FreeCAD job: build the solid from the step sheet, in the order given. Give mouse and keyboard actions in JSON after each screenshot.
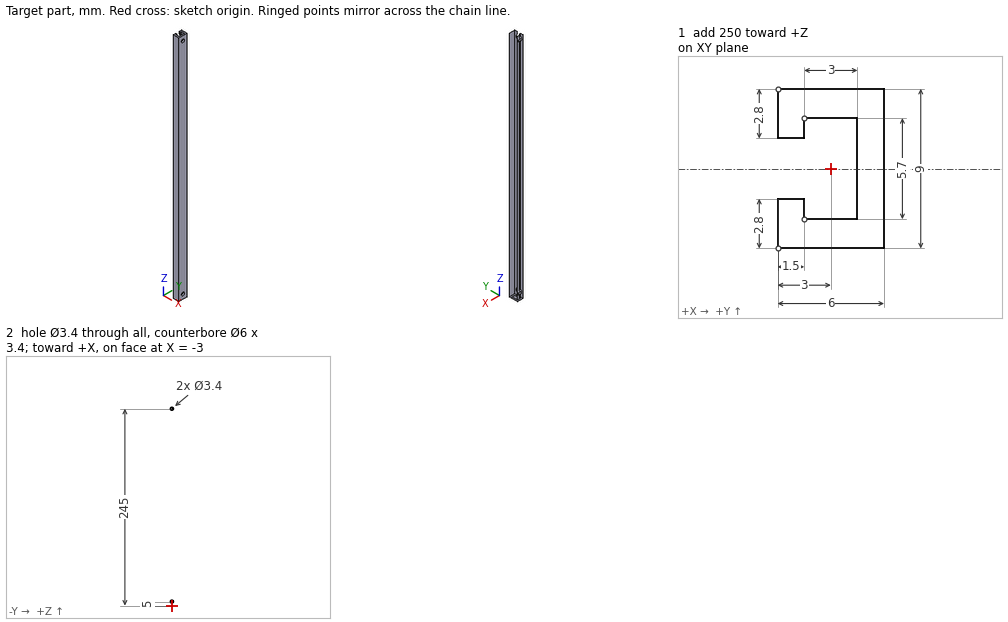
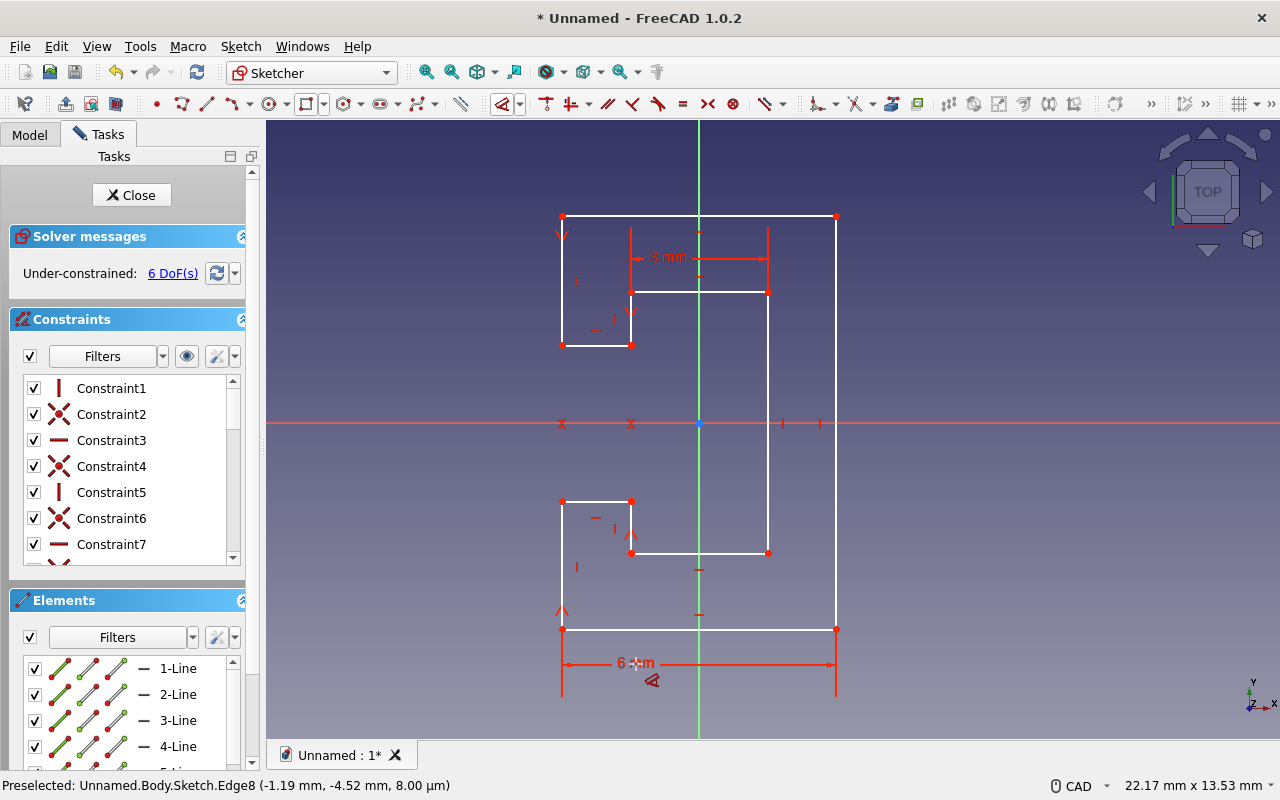
{"action": "left_click", "coordinate": [836, 506]}
{"action": "left_click", "coordinate": [870, 328]}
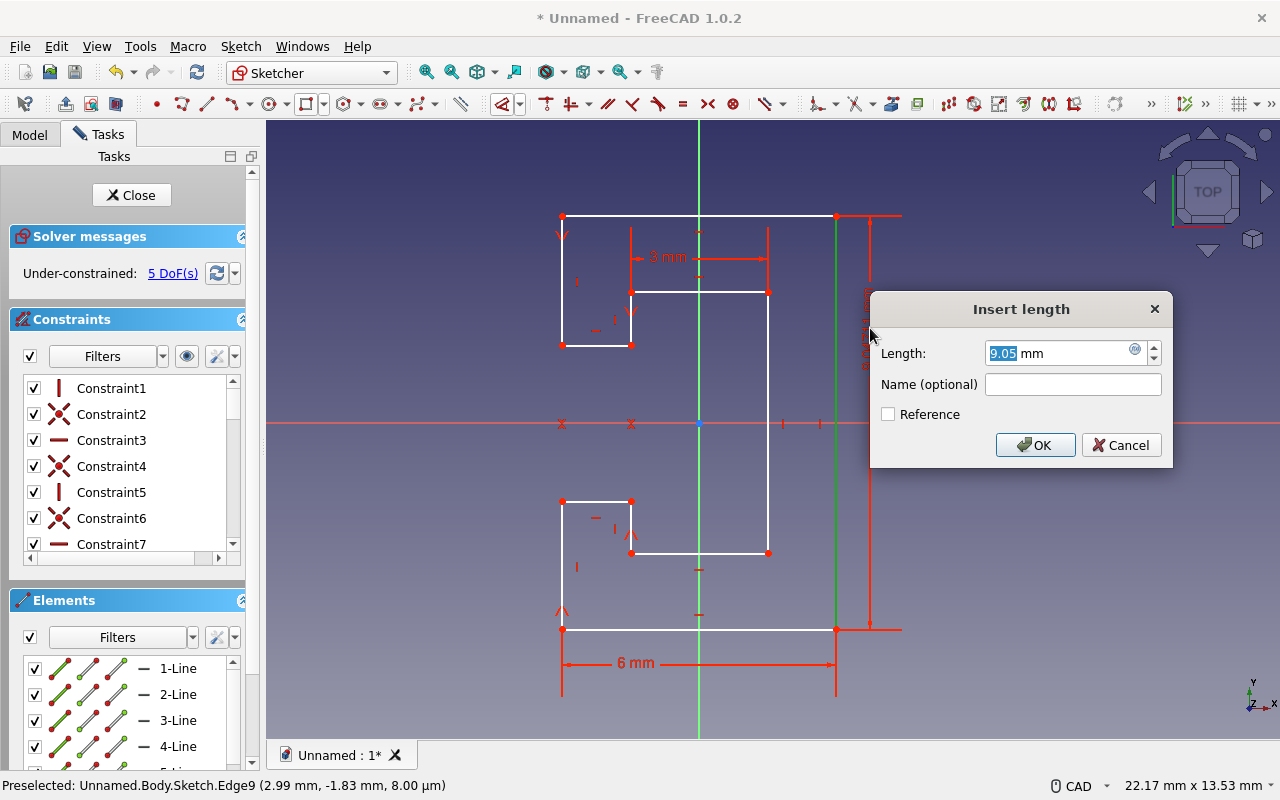
{"action": "type", "text": "9"}
{"action": "key", "text": "Return"}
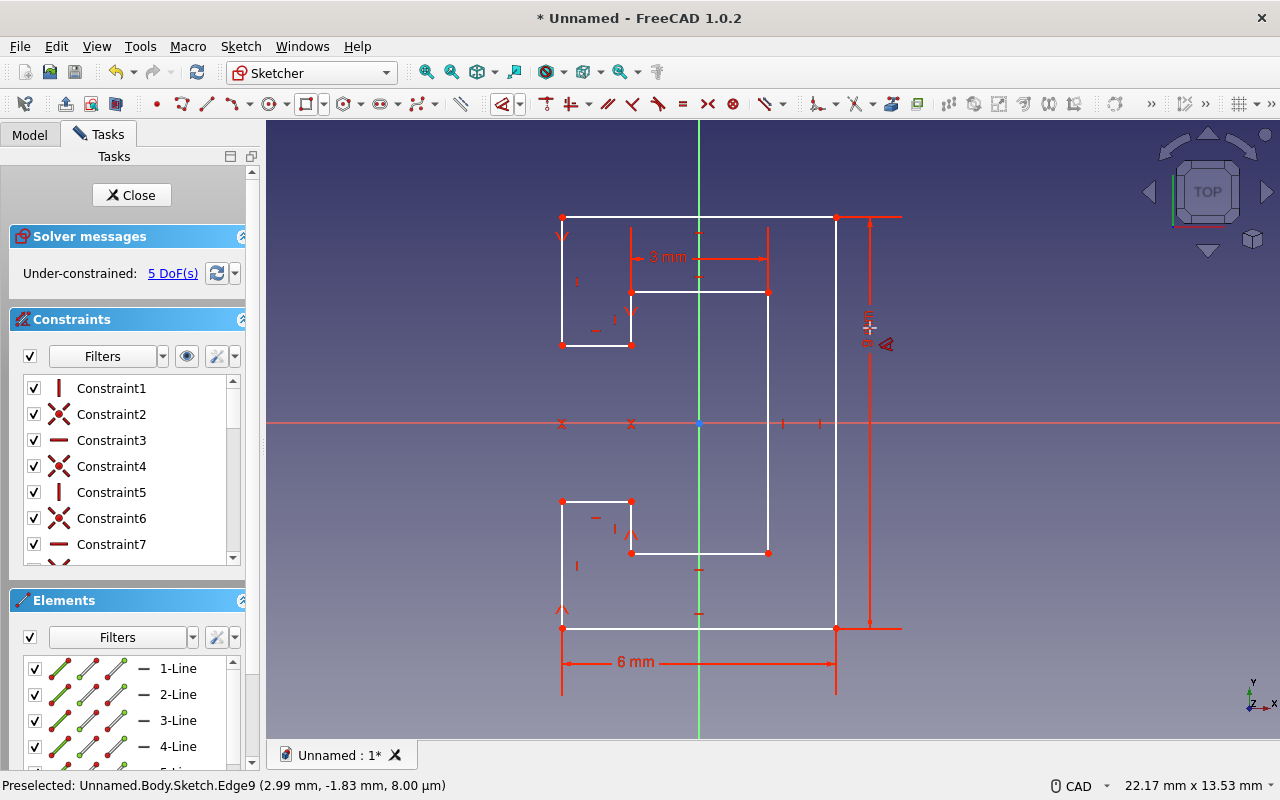
{"action": "left_click", "coordinate": [562, 502]}
{"action": "left_click", "coordinate": [599, 536]}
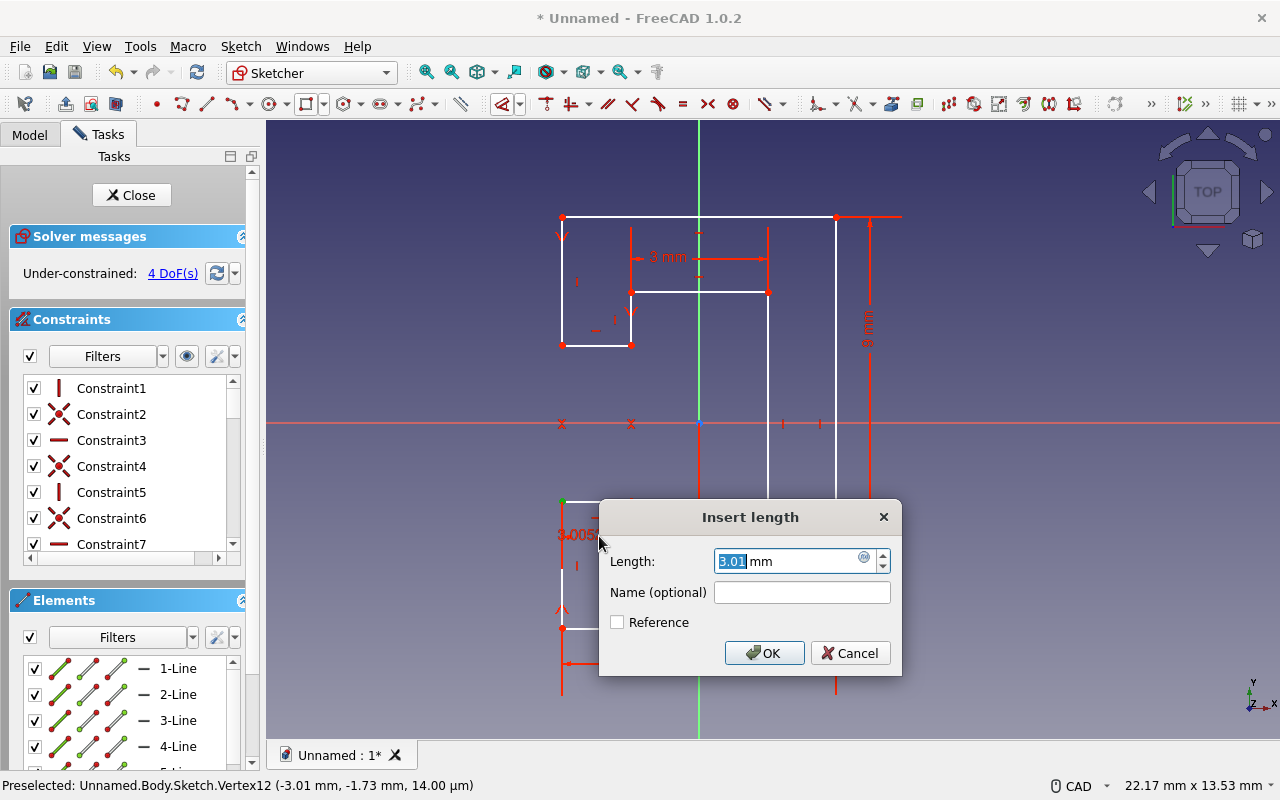
{"action": "type", "text": "3"}
{"action": "key", "text": "Return"}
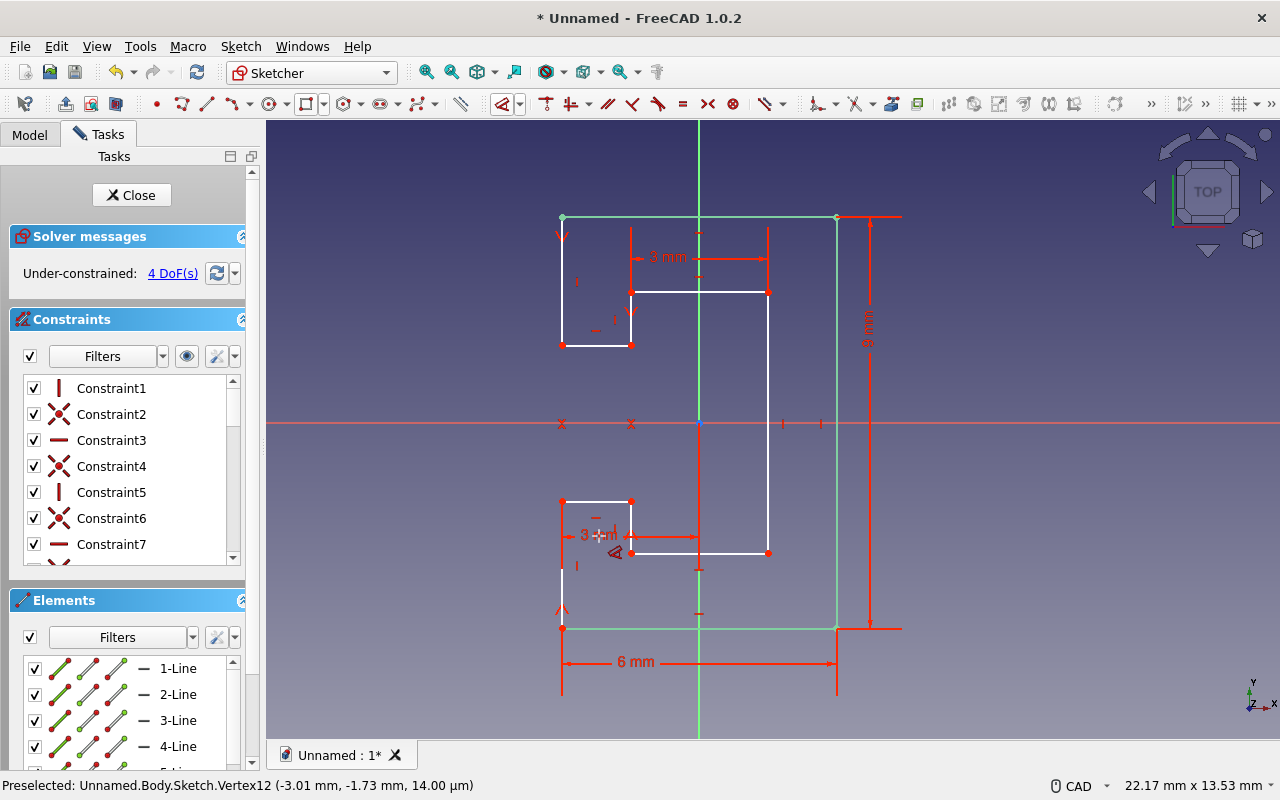
{"action": "left_click", "coordinate": [768, 371]}
{"action": "left_click", "coordinate": [802, 363]}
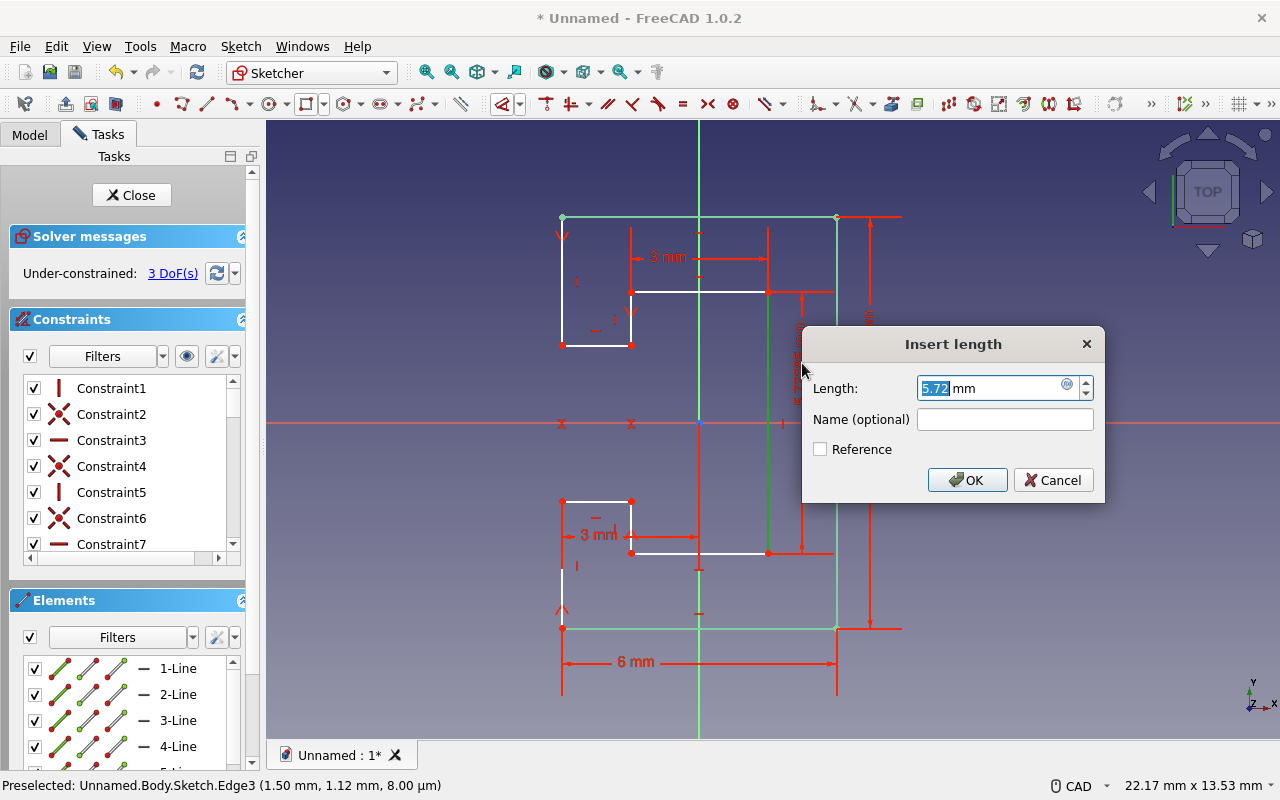
{"action": "type", "text": "5.7"}
{"action": "key", "text": "Return"}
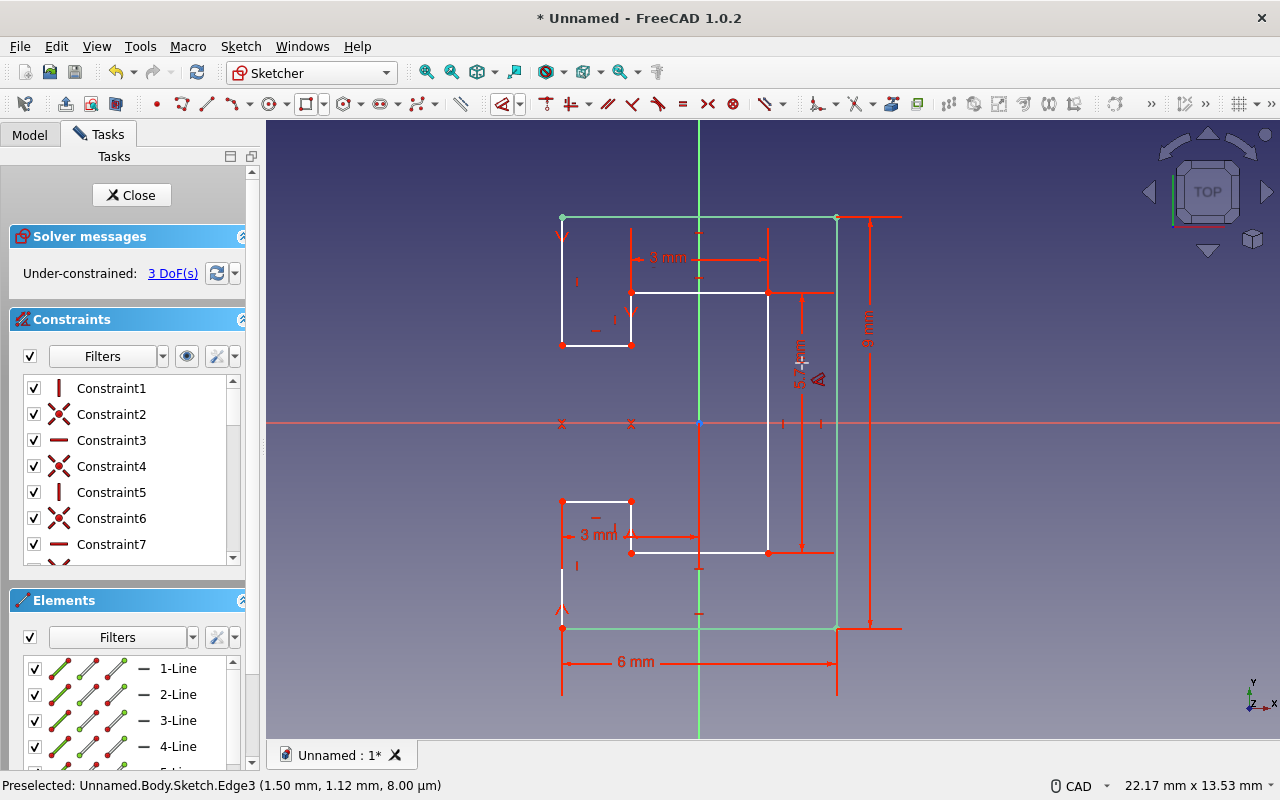
{"action": "left_click", "coordinate": [610, 502]}
{"action": "left_click", "coordinate": [597, 468]}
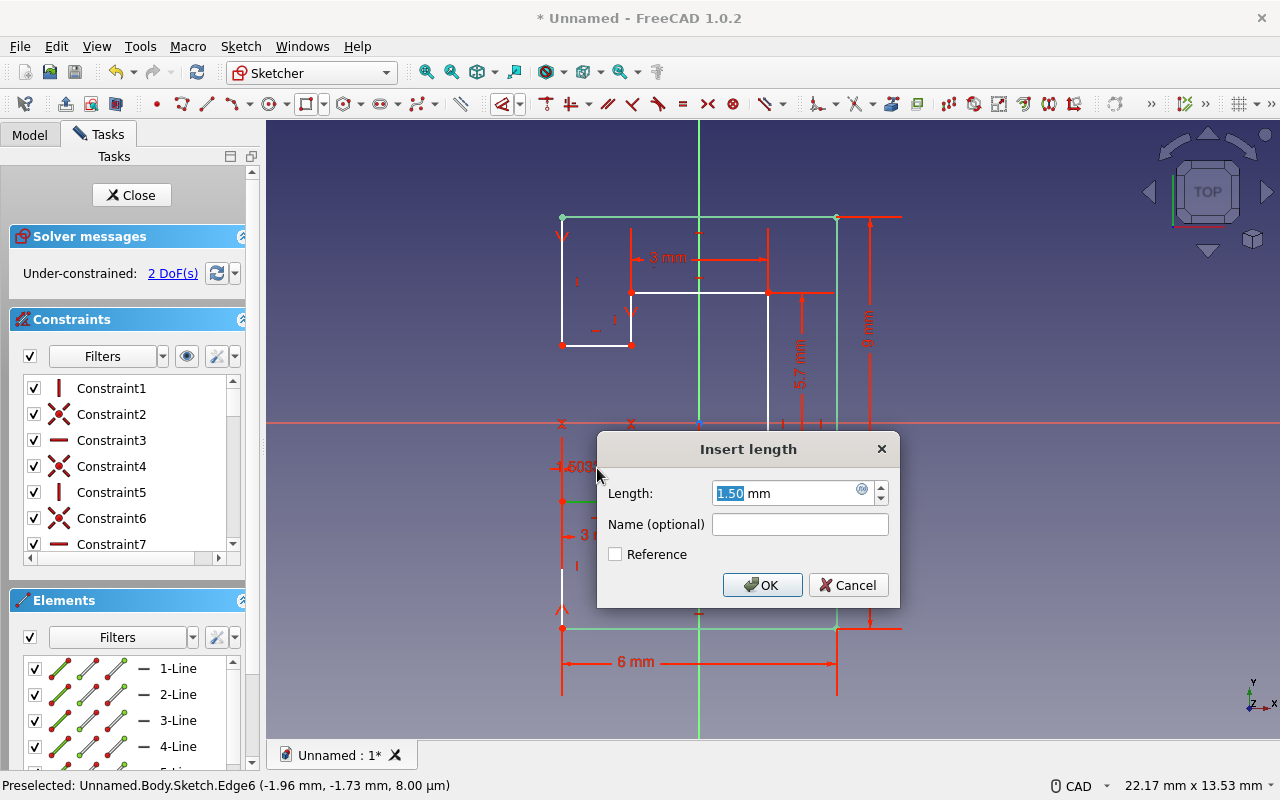
{"action": "type", "text": "1.5"}
{"action": "key", "text": "Return"}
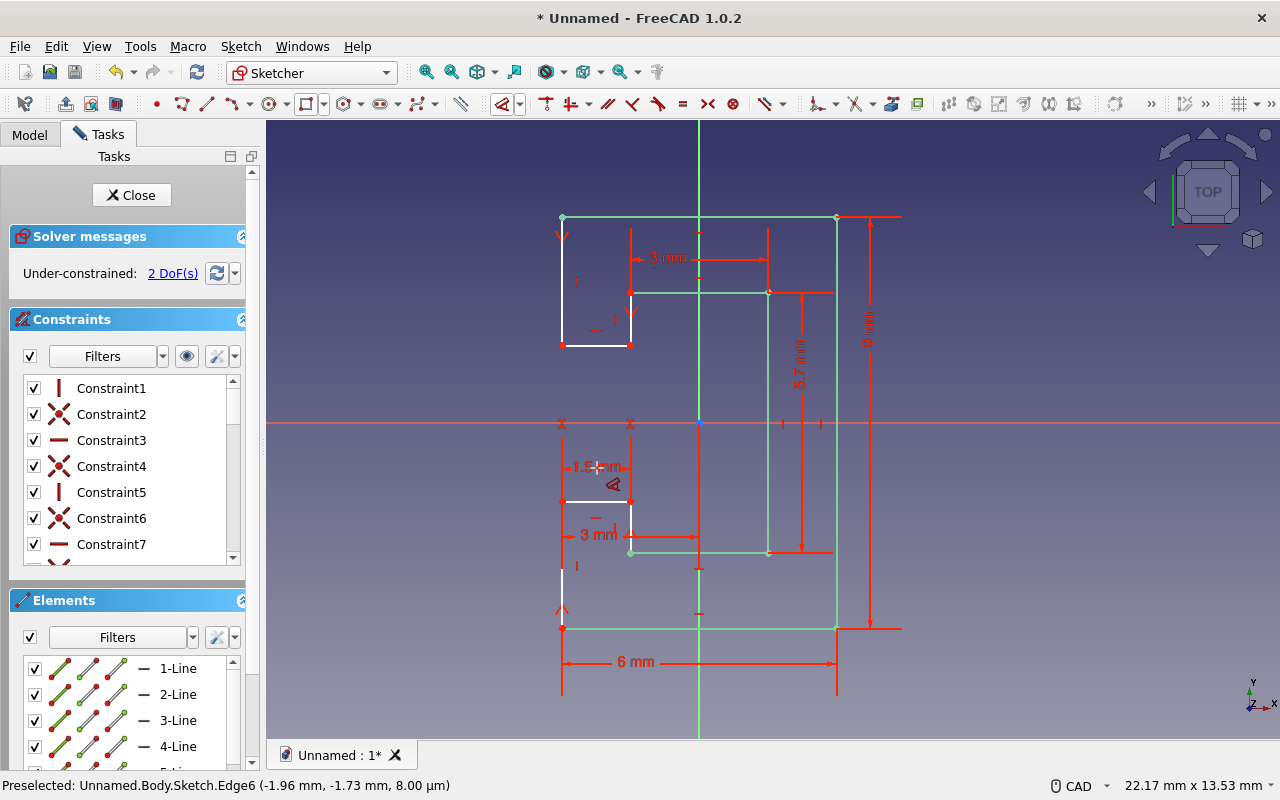
{"action": "left_click", "coordinate": [562, 540]}
{"action": "left_click", "coordinate": [528, 565]}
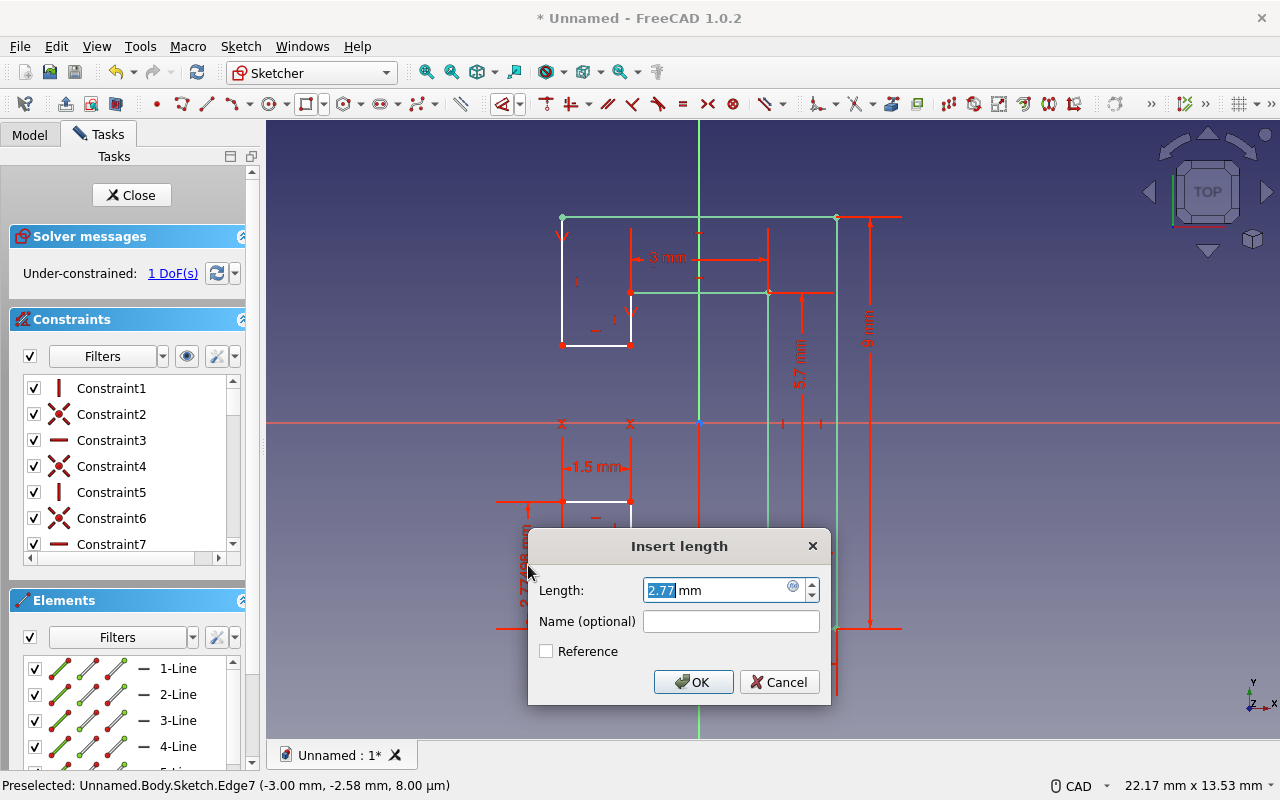
{"action": "type", "text": "2.8"}
{"action": "key", "text": "Return"}